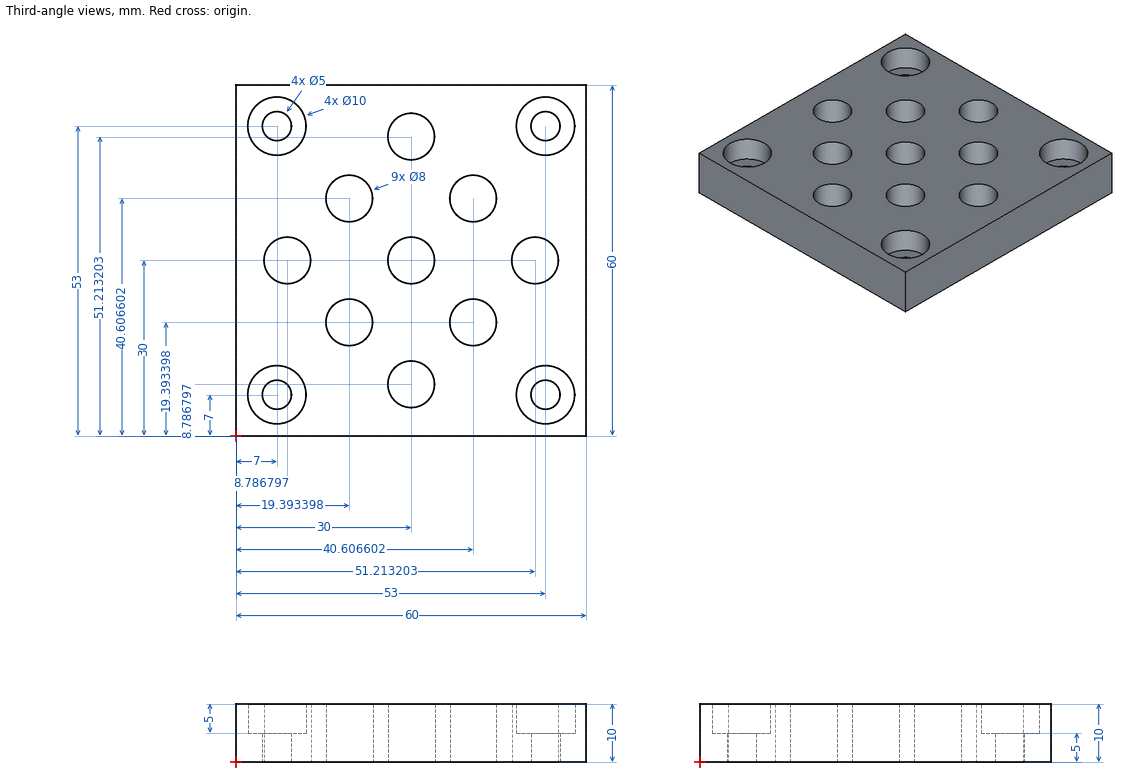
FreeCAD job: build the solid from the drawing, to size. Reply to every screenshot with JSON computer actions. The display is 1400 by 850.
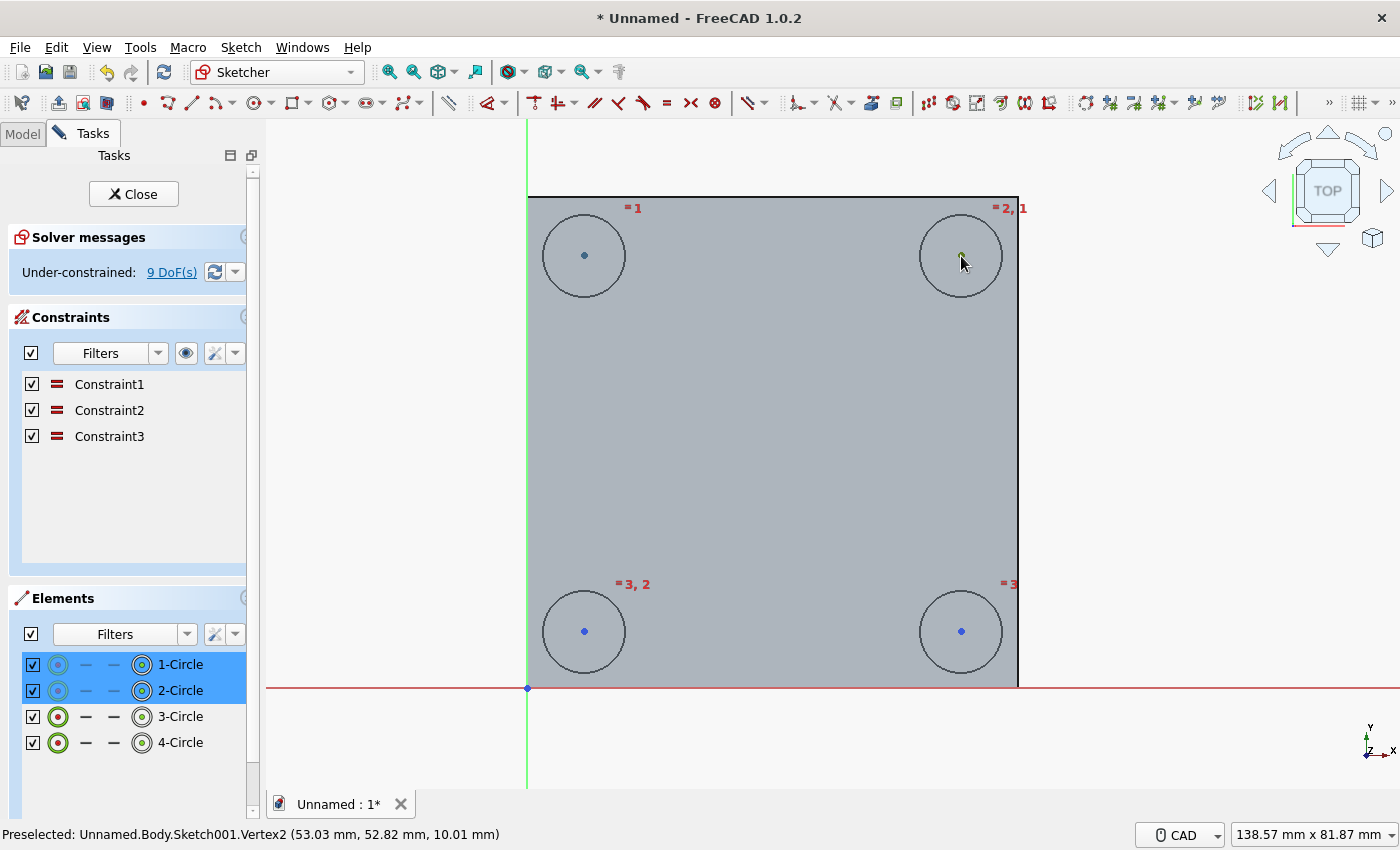
{"action": "key", "text": "h"}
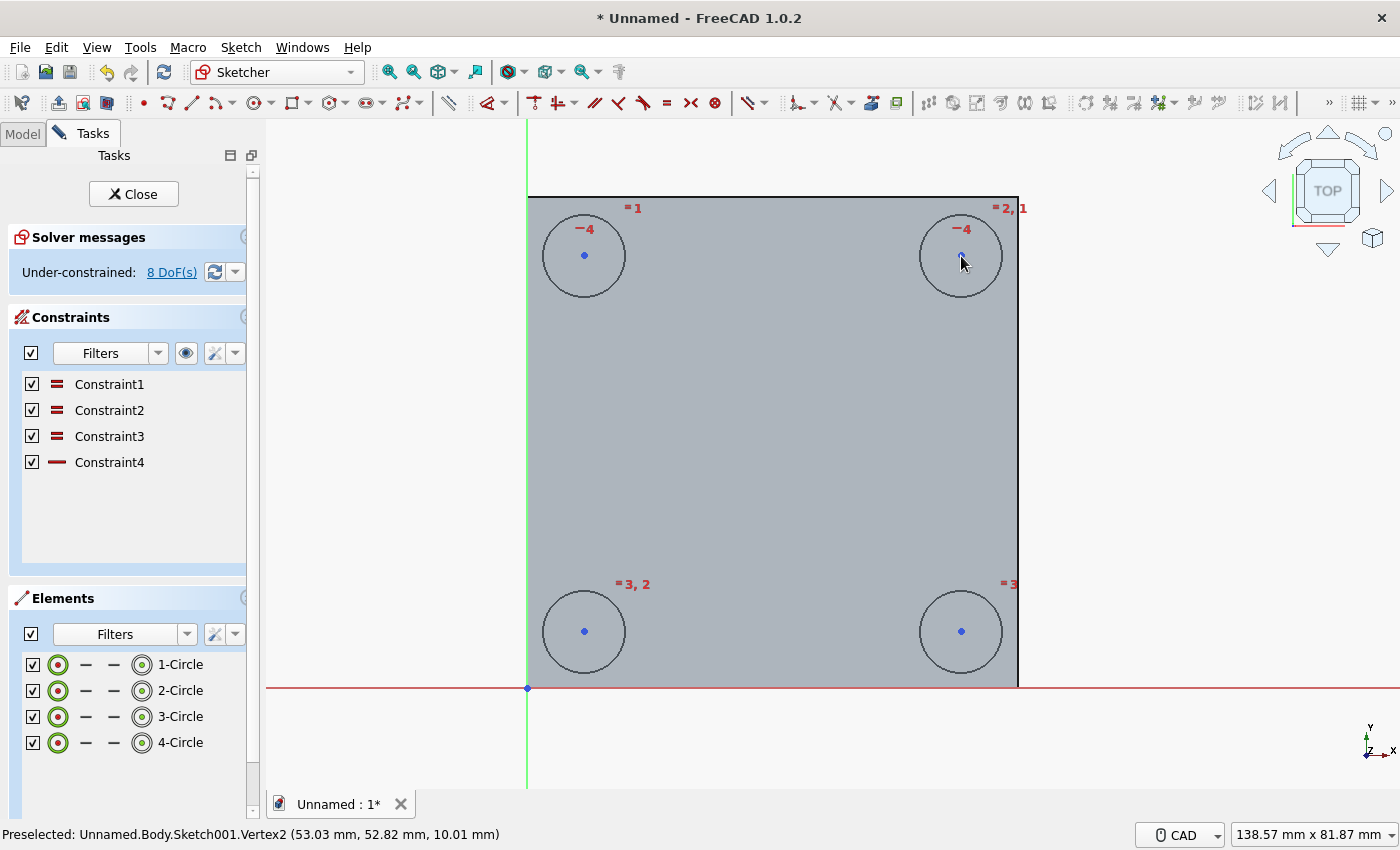
{"action": "left_click", "coordinate": [584, 256]}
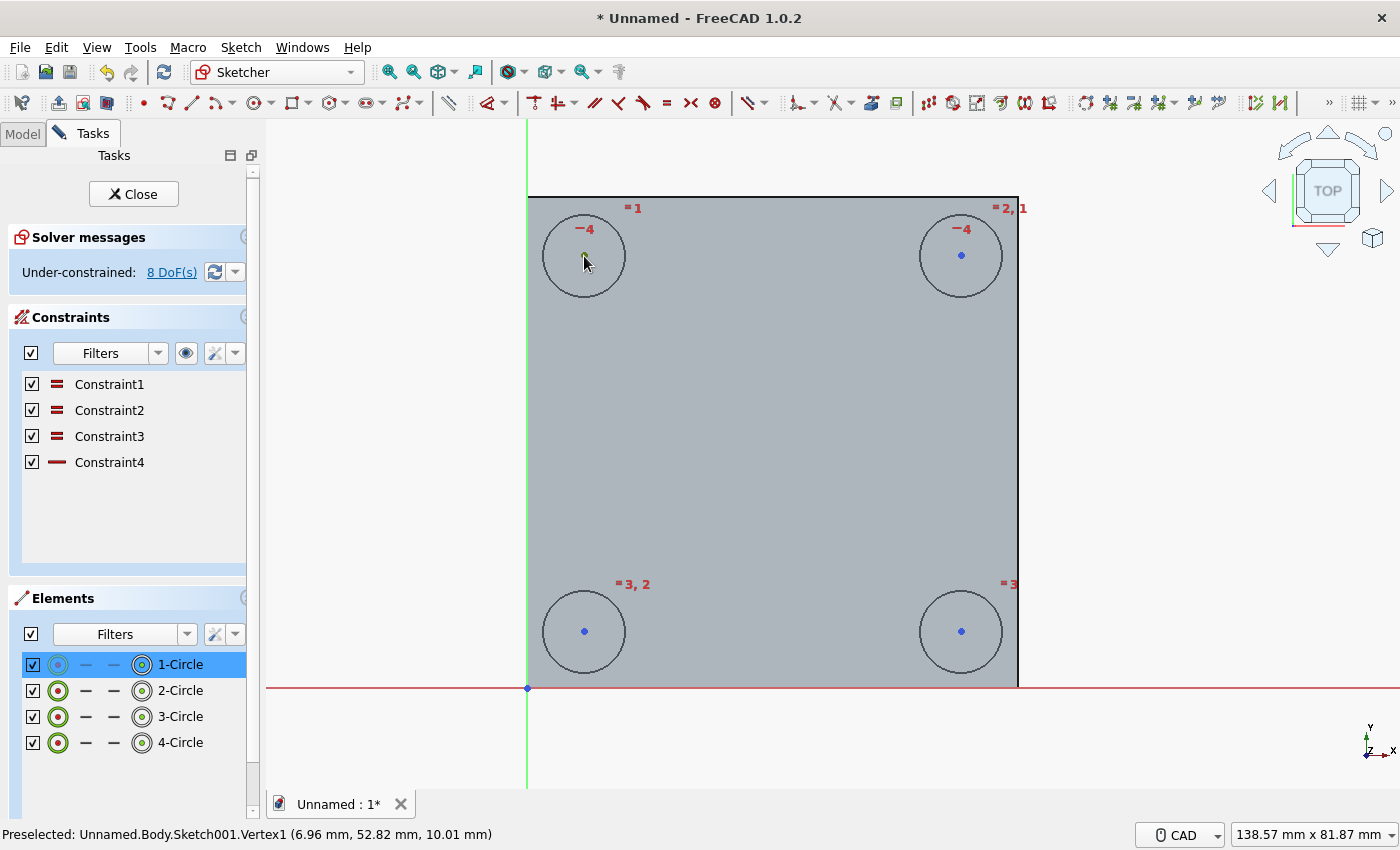
{"action": "left_click", "coordinate": [584, 632]}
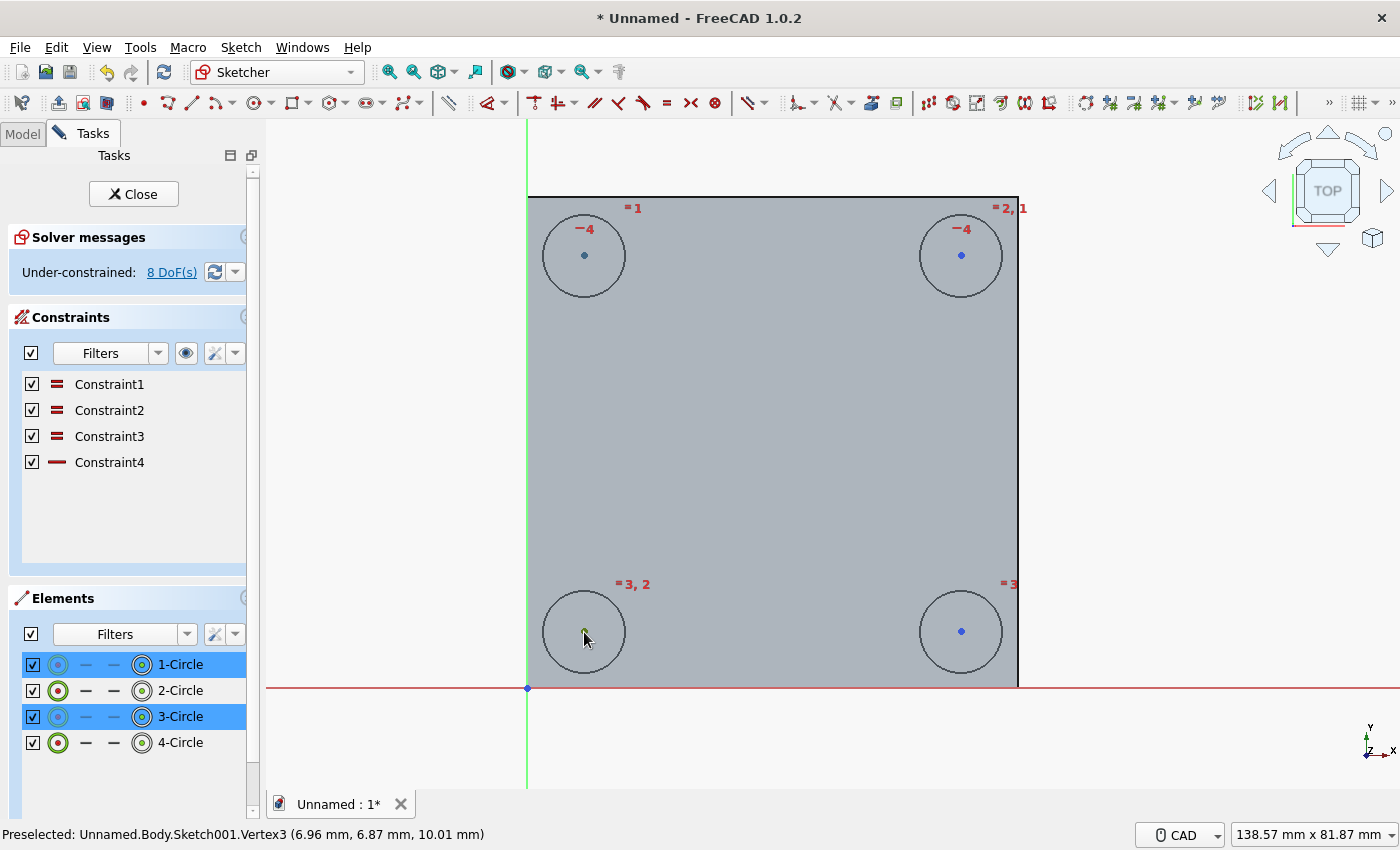
{"action": "key", "text": "v"}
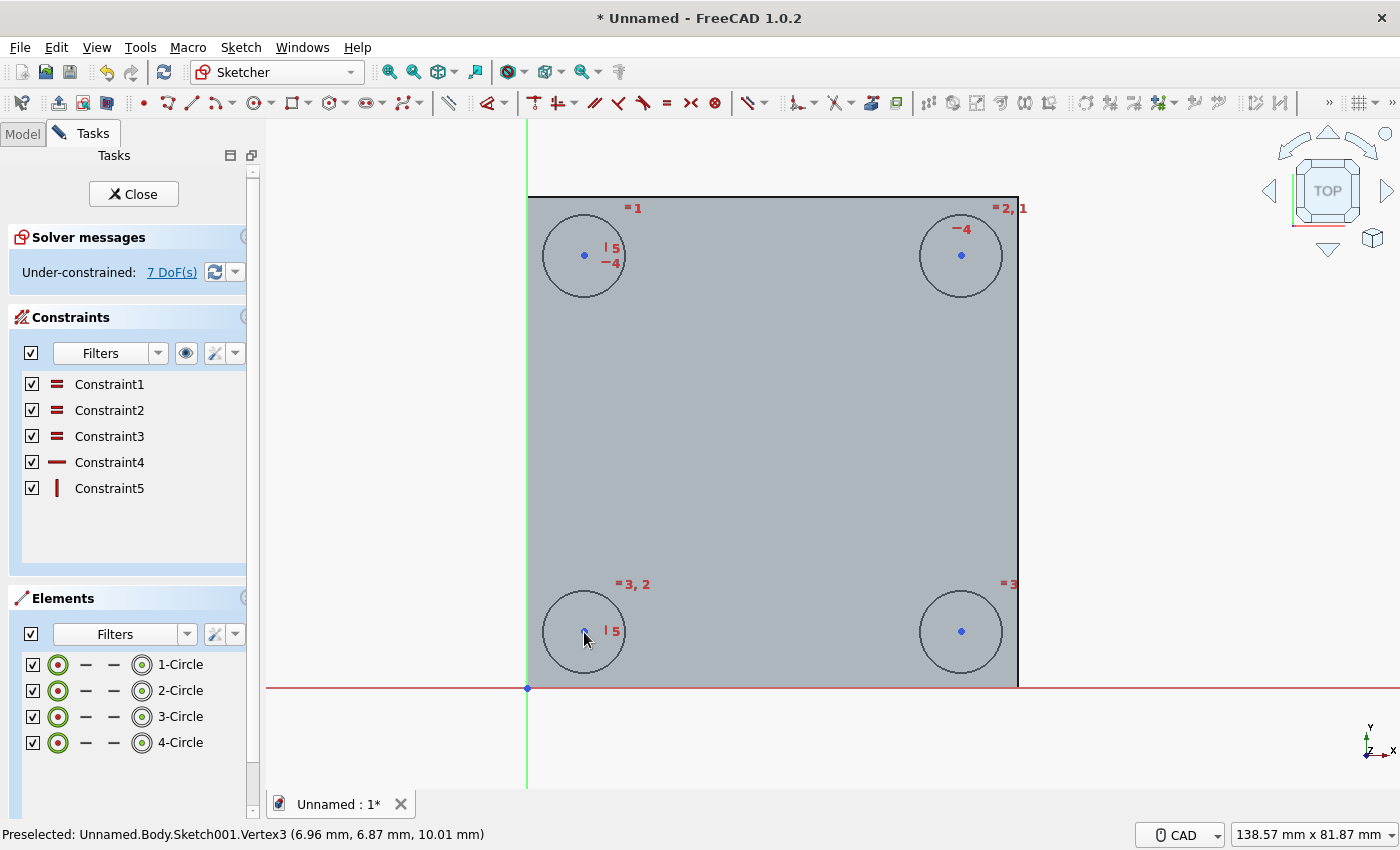
{"action": "left_click", "coordinate": [961, 256]}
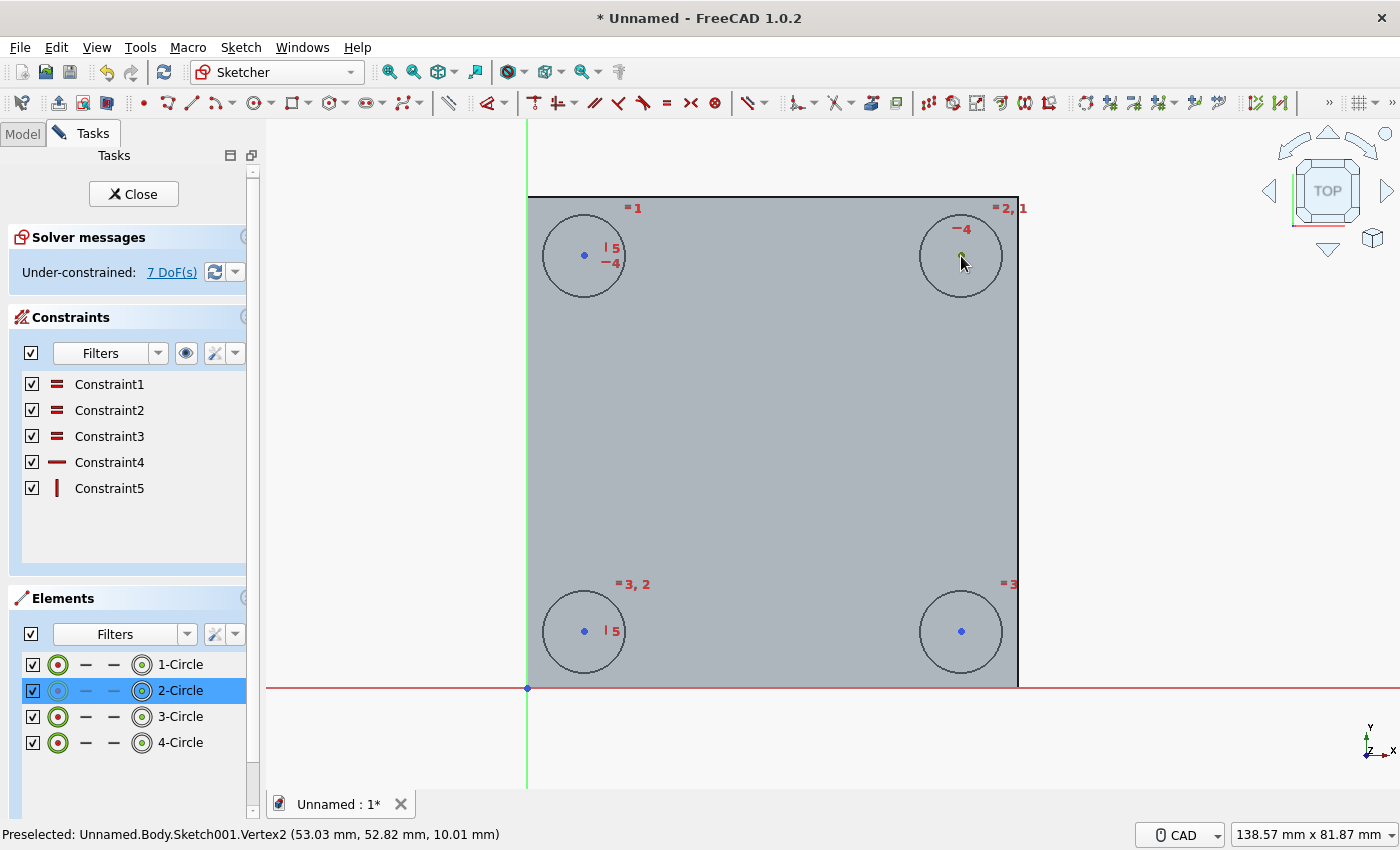
{"action": "left_click", "coordinate": [961, 632]}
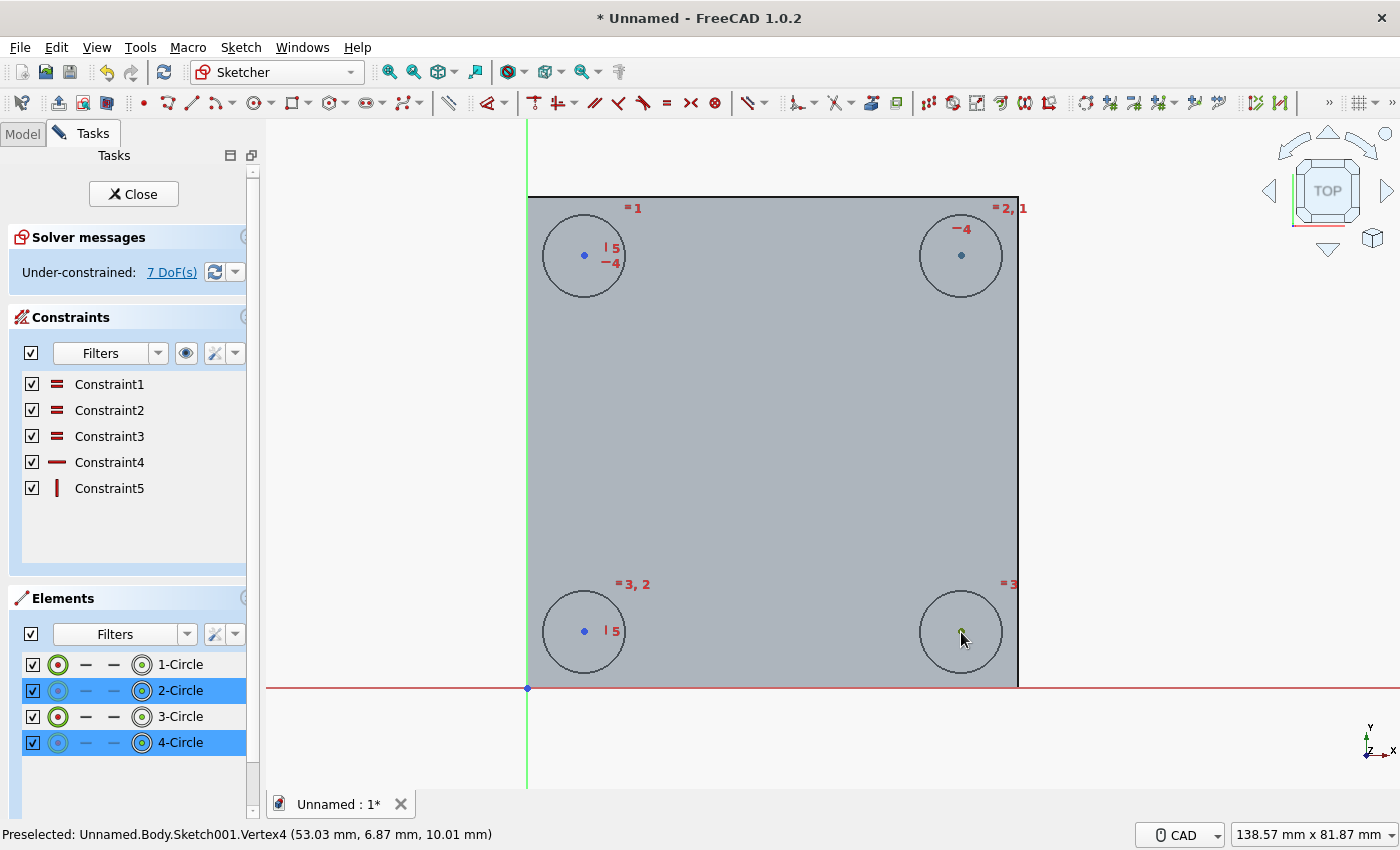
{"action": "key", "text": "v"}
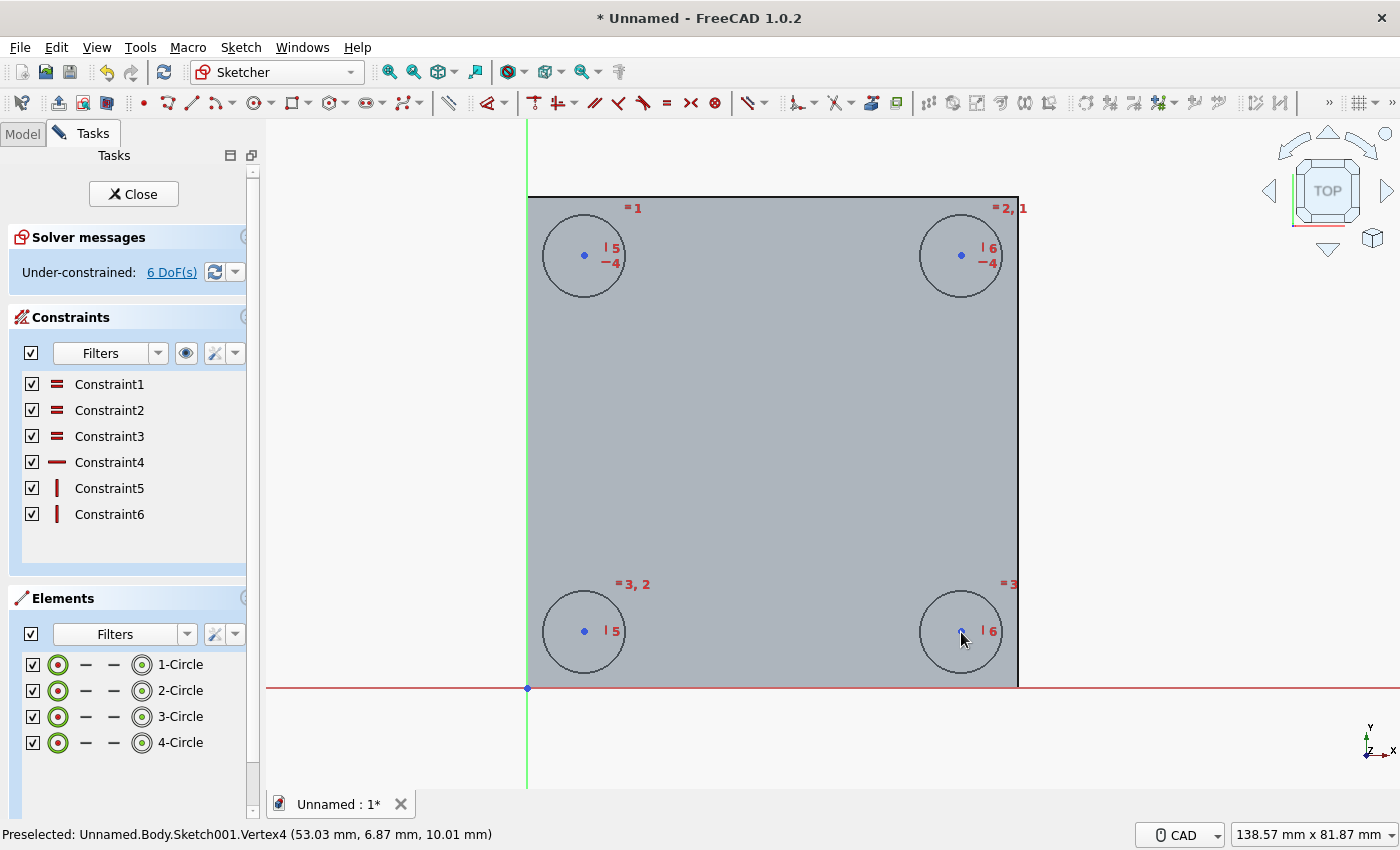
{"action": "left_click", "coordinate": [584, 632]}